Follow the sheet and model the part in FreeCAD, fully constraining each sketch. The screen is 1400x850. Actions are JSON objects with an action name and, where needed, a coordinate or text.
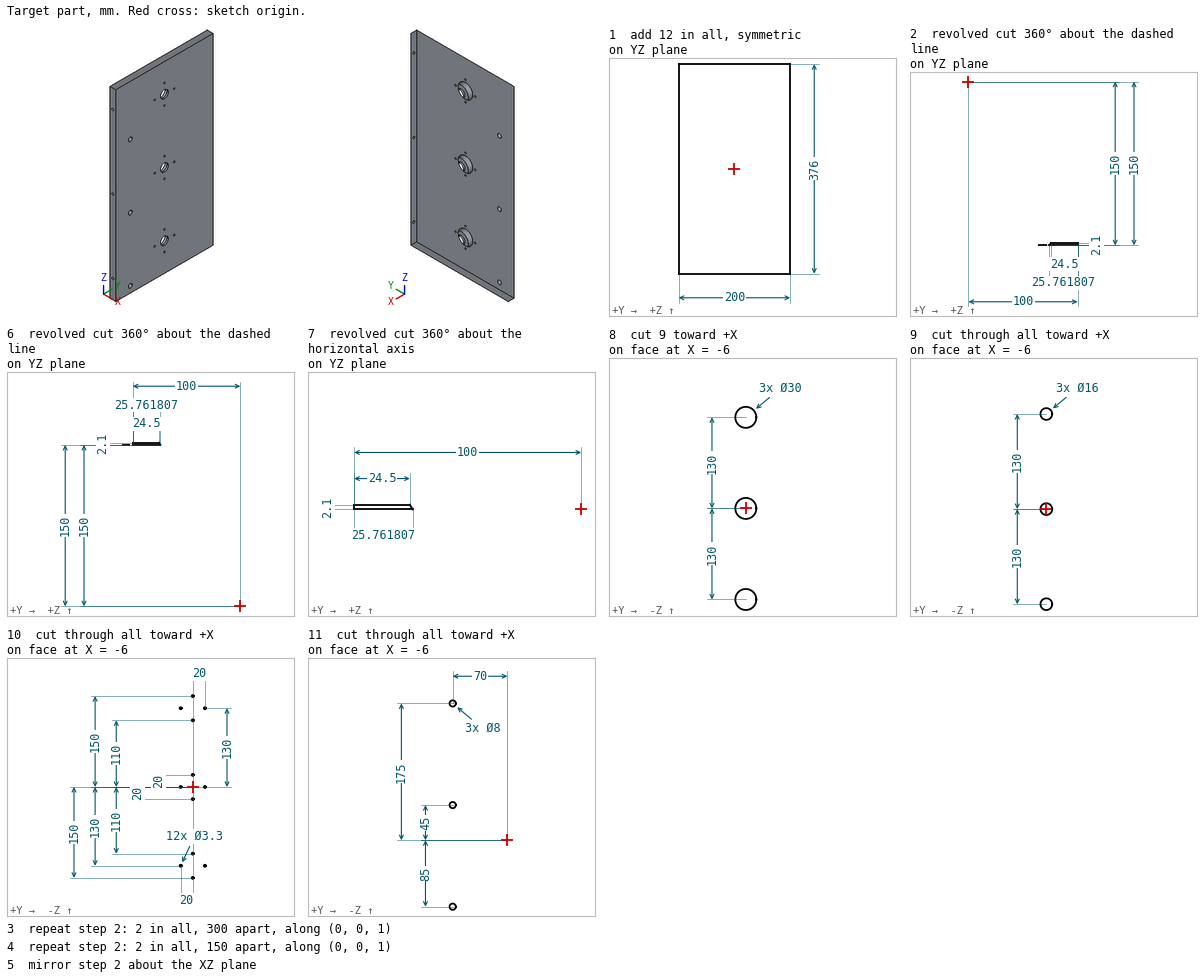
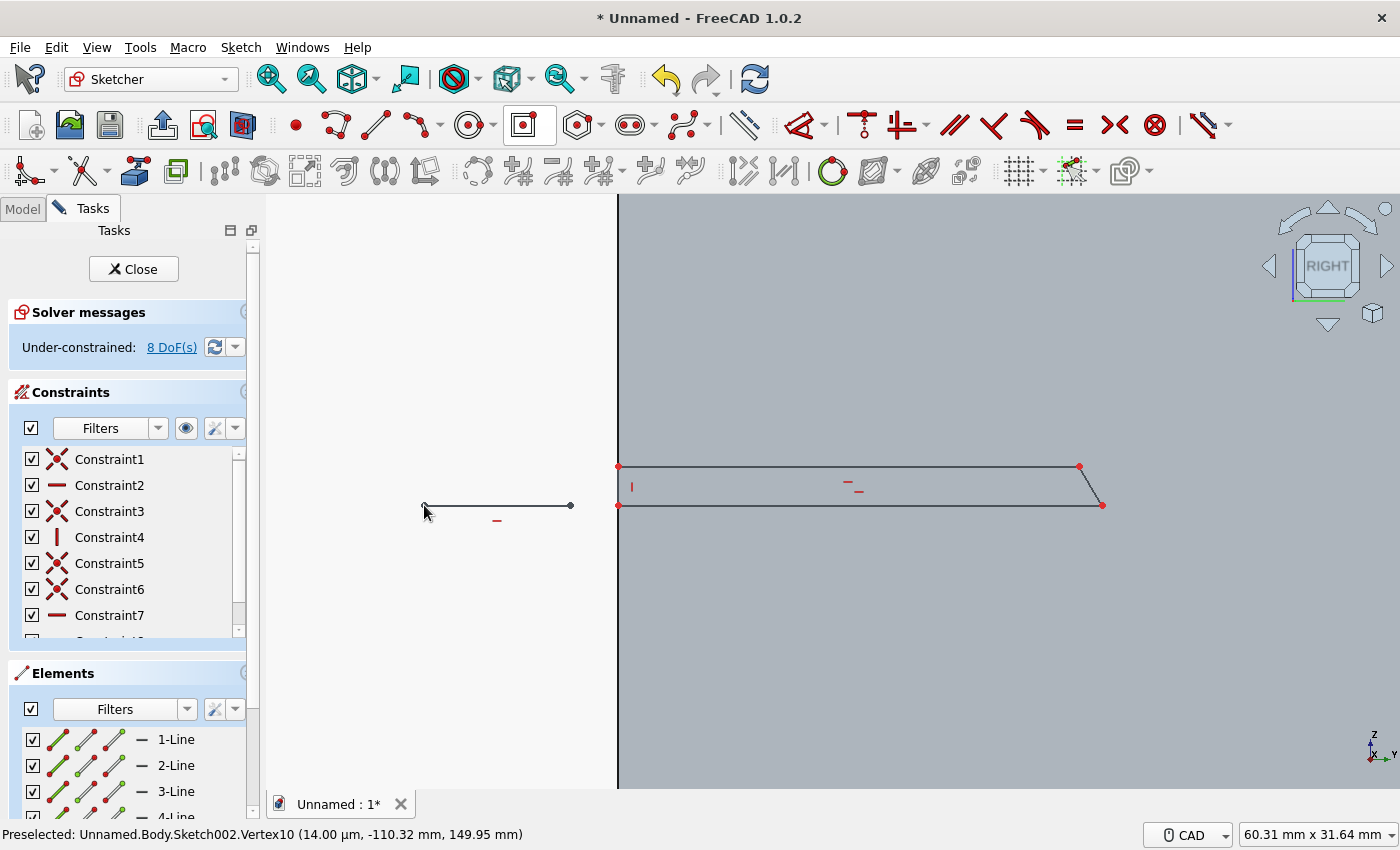
{"action": "left_click", "coordinate": [526, 506]}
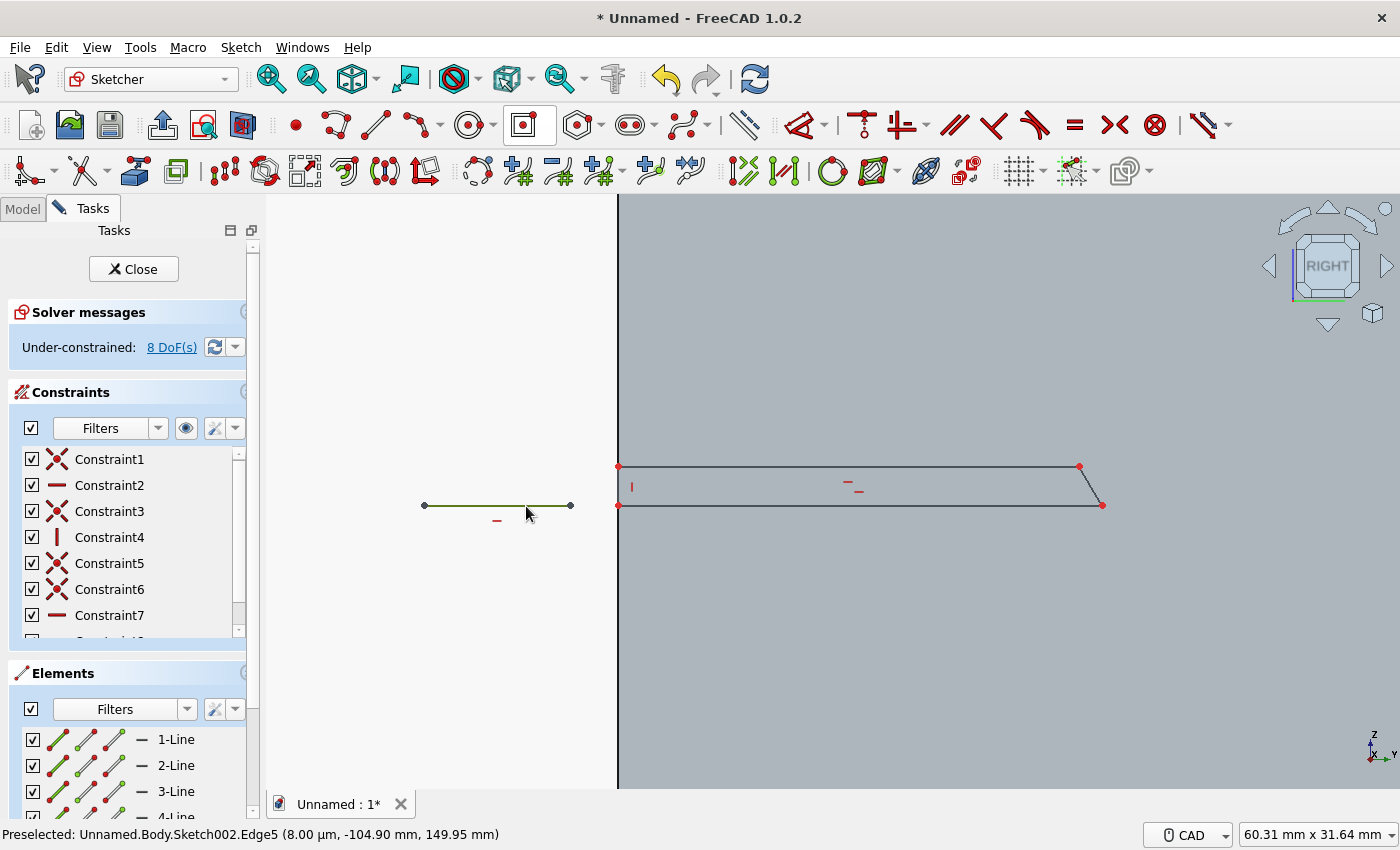
{"action": "left_click", "coordinate": [746, 126]}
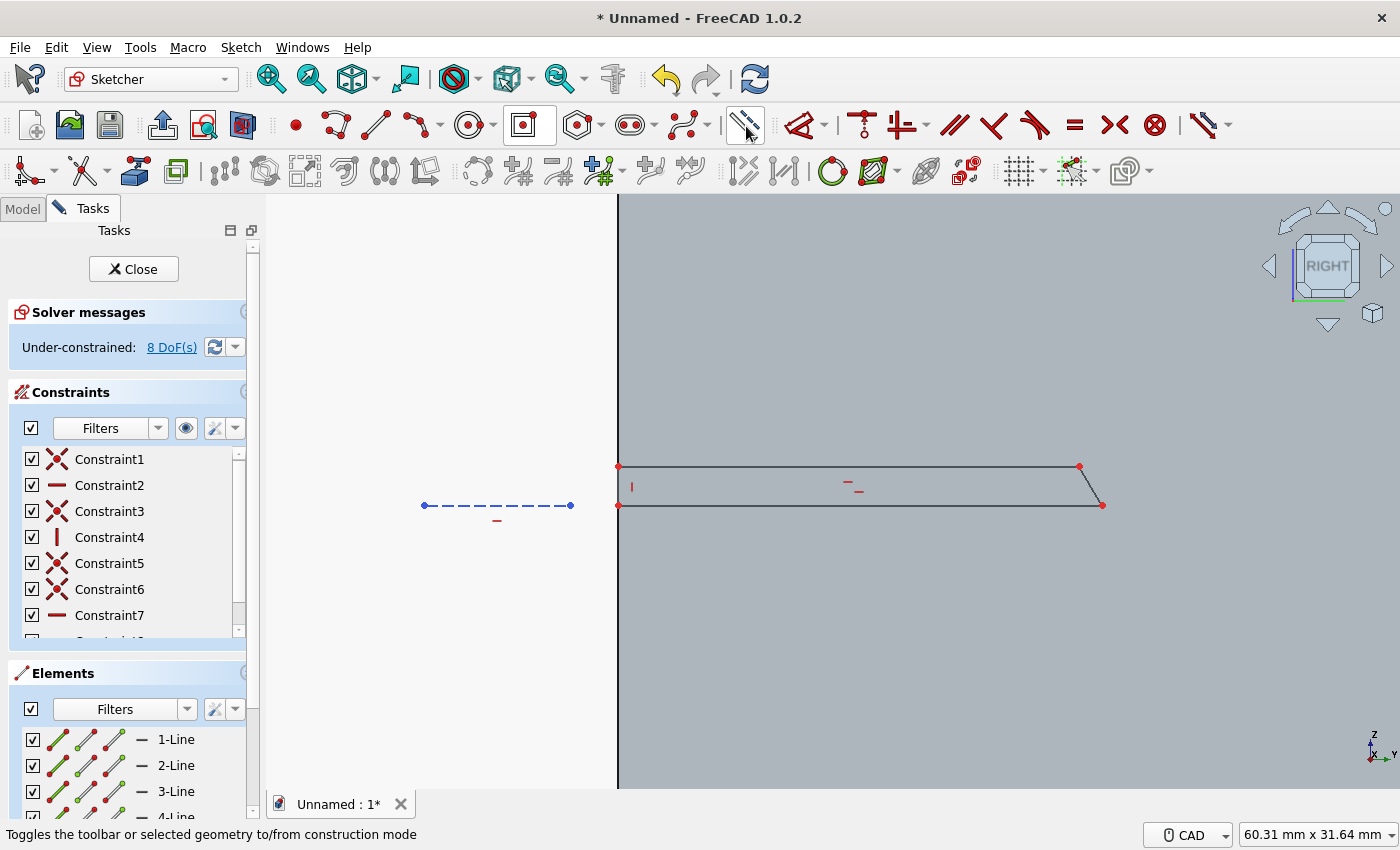
{"action": "left_click", "coordinate": [800, 126]}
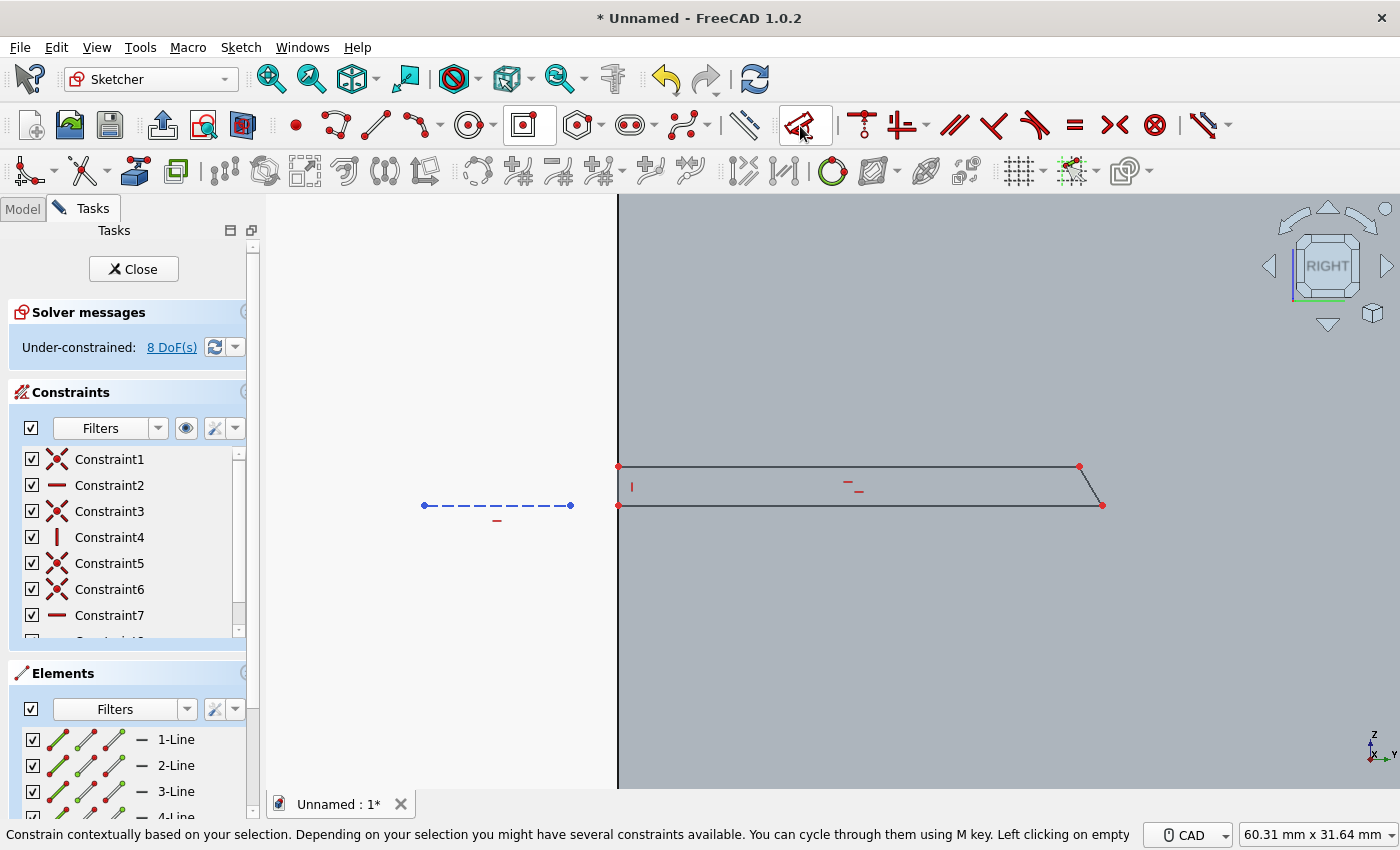
{"action": "left_click", "coordinate": [618, 479]}
{"action": "left_click", "coordinate": [584, 486]}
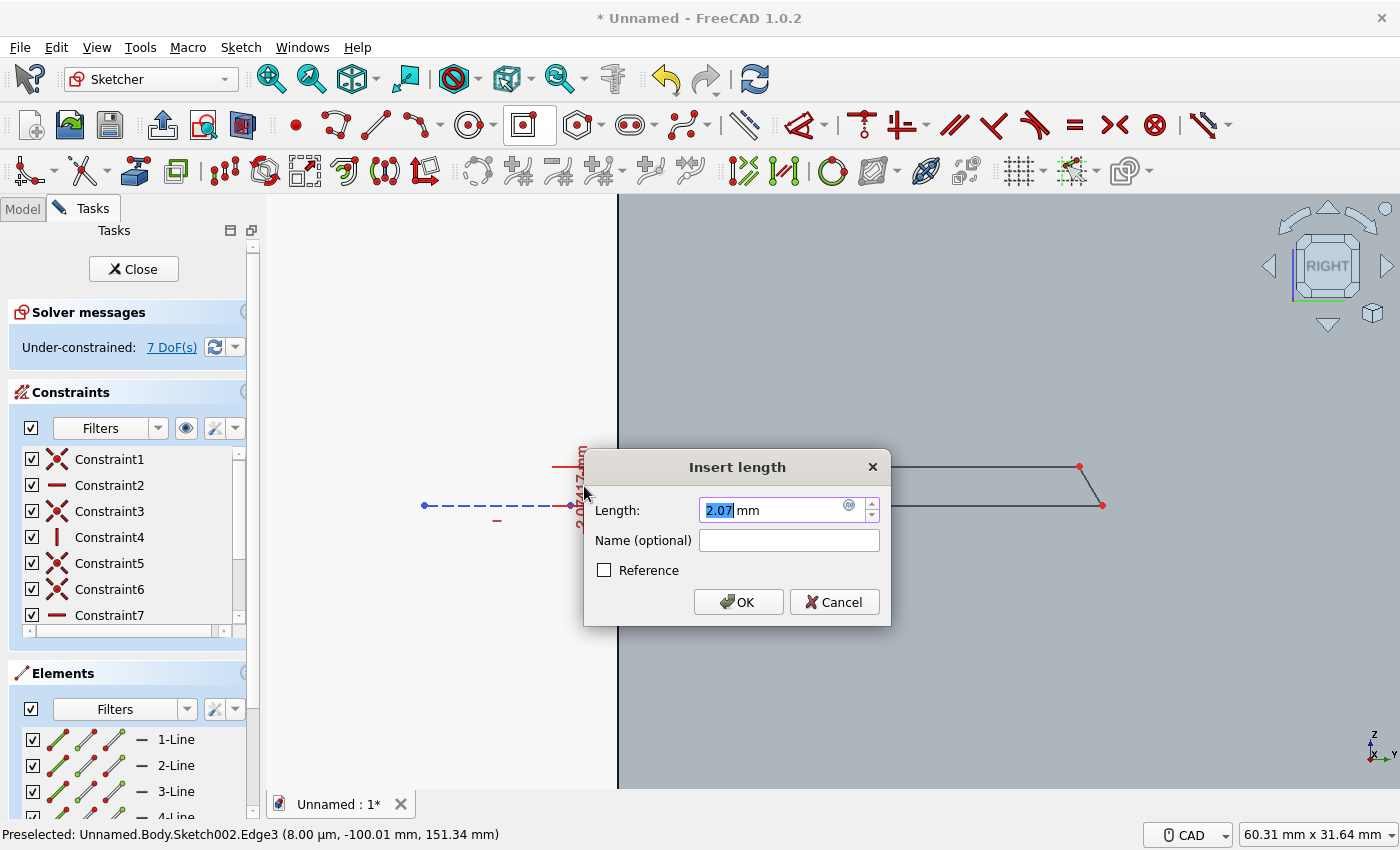
{"action": "type", "text": "2.1"}
{"action": "key", "text": "Return"}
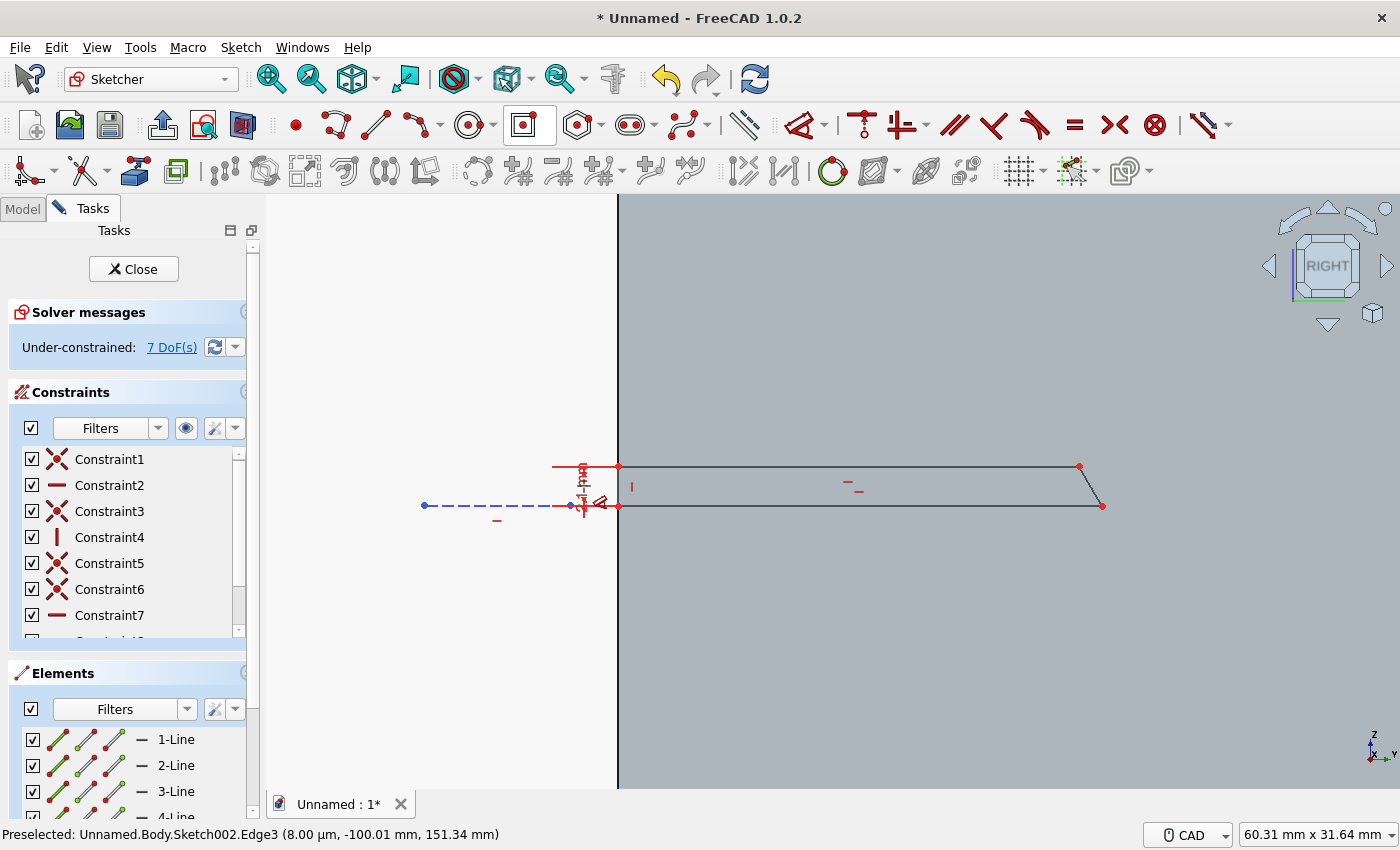
{"action": "left_click", "coordinate": [941, 467]}
{"action": "left_click", "coordinate": [848, 433]}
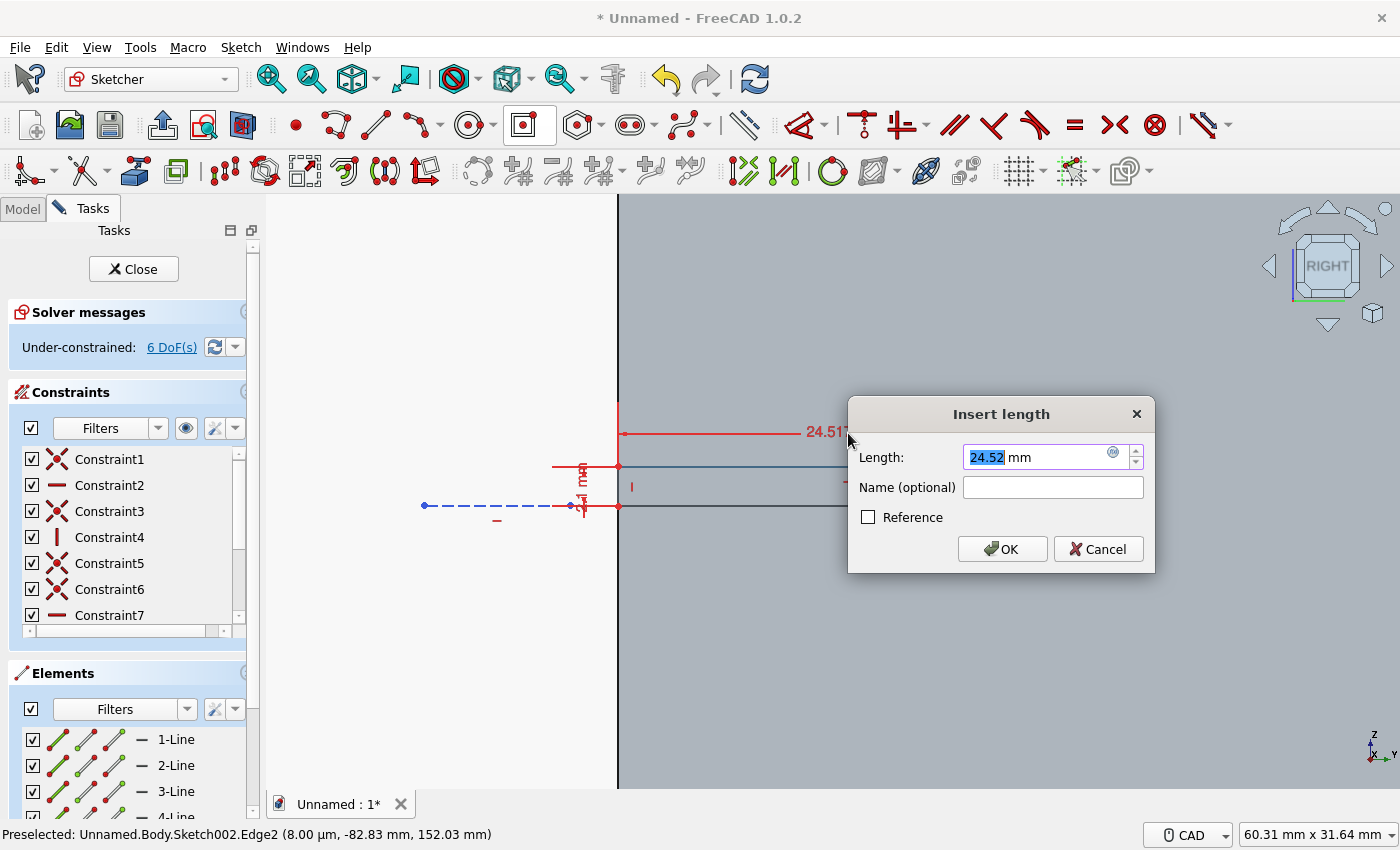
{"action": "type", "text": "24.5"}
{"action": "key", "text": "Return"}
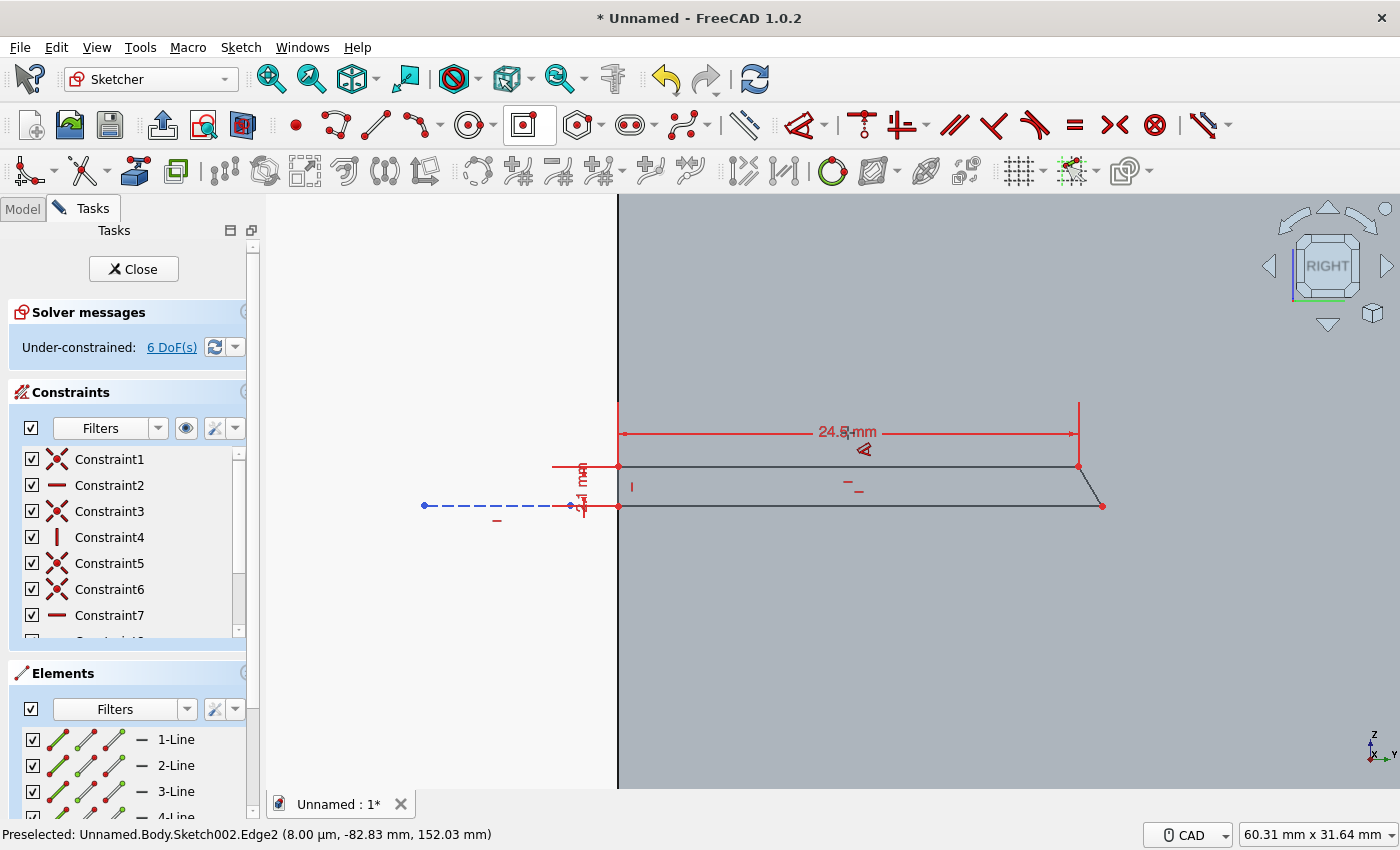
{"action": "left_click", "coordinate": [1102, 506]}
{"action": "left_click", "coordinate": [1068, 634]}